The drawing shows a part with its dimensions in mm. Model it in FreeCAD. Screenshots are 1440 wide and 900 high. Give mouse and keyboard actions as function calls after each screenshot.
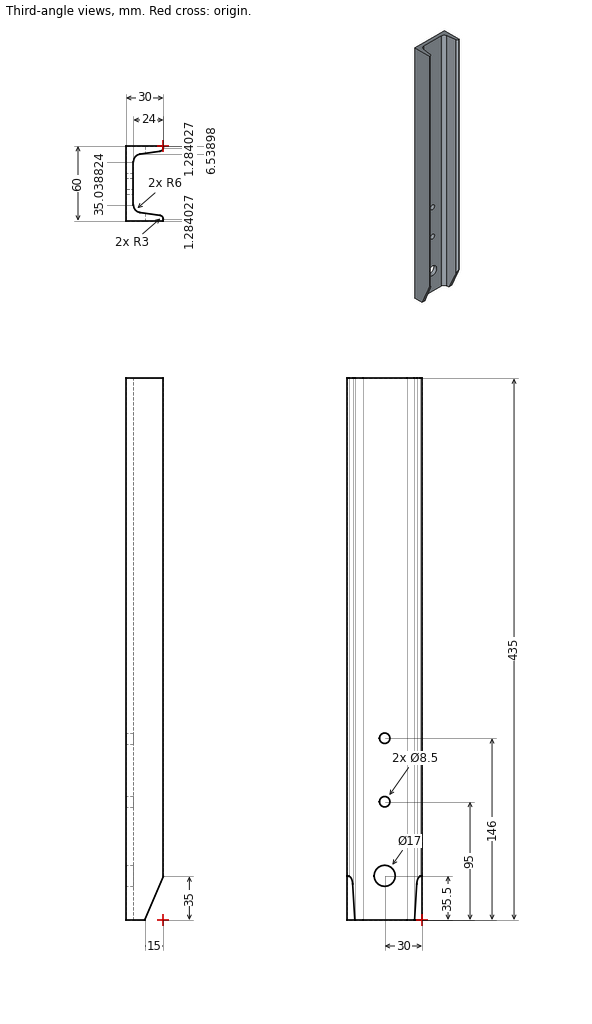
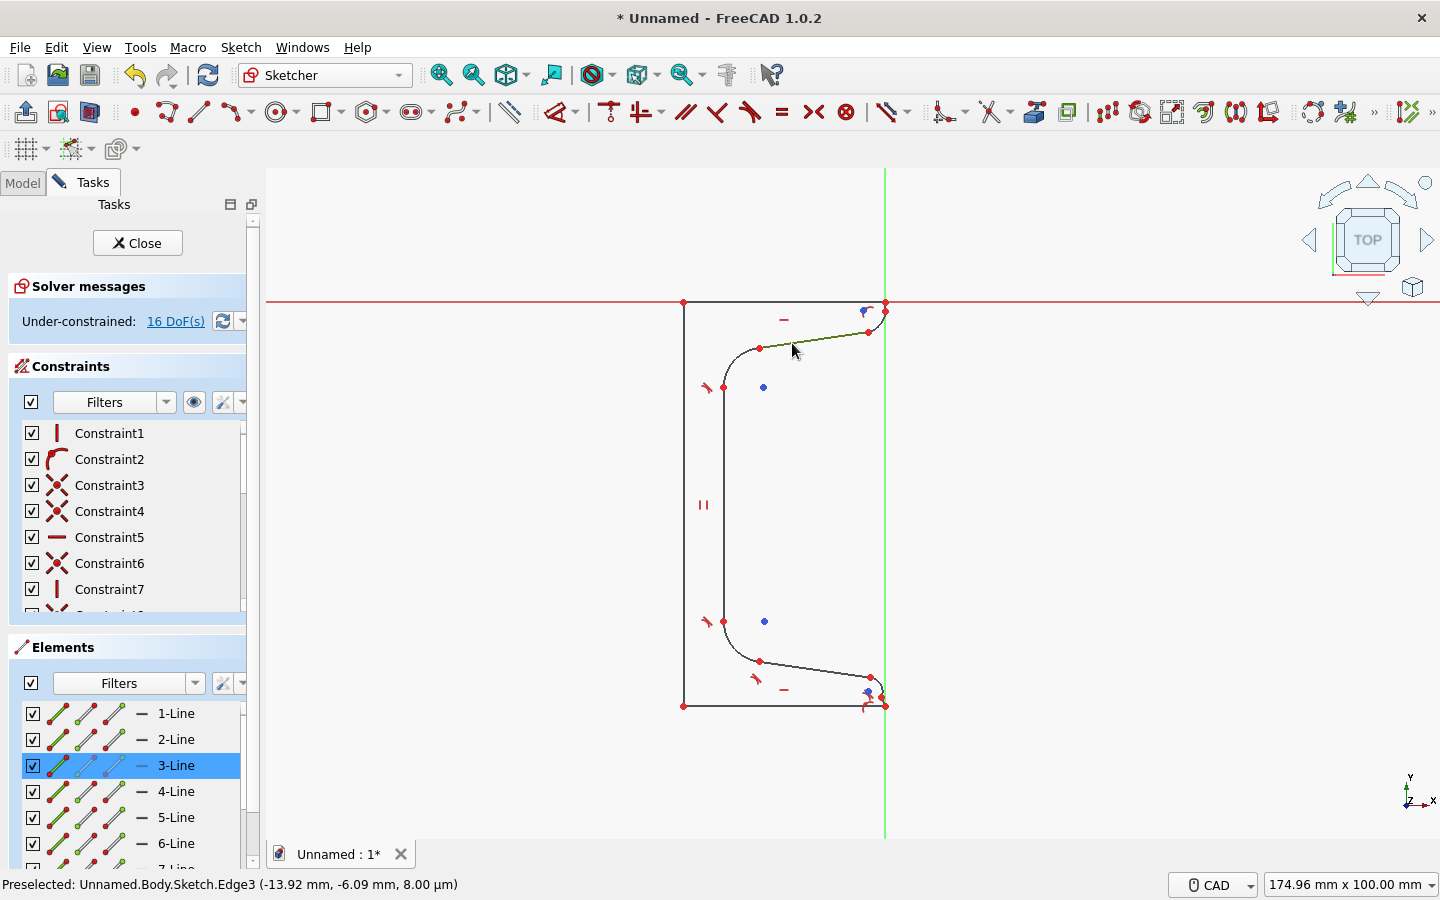
click(743, 353)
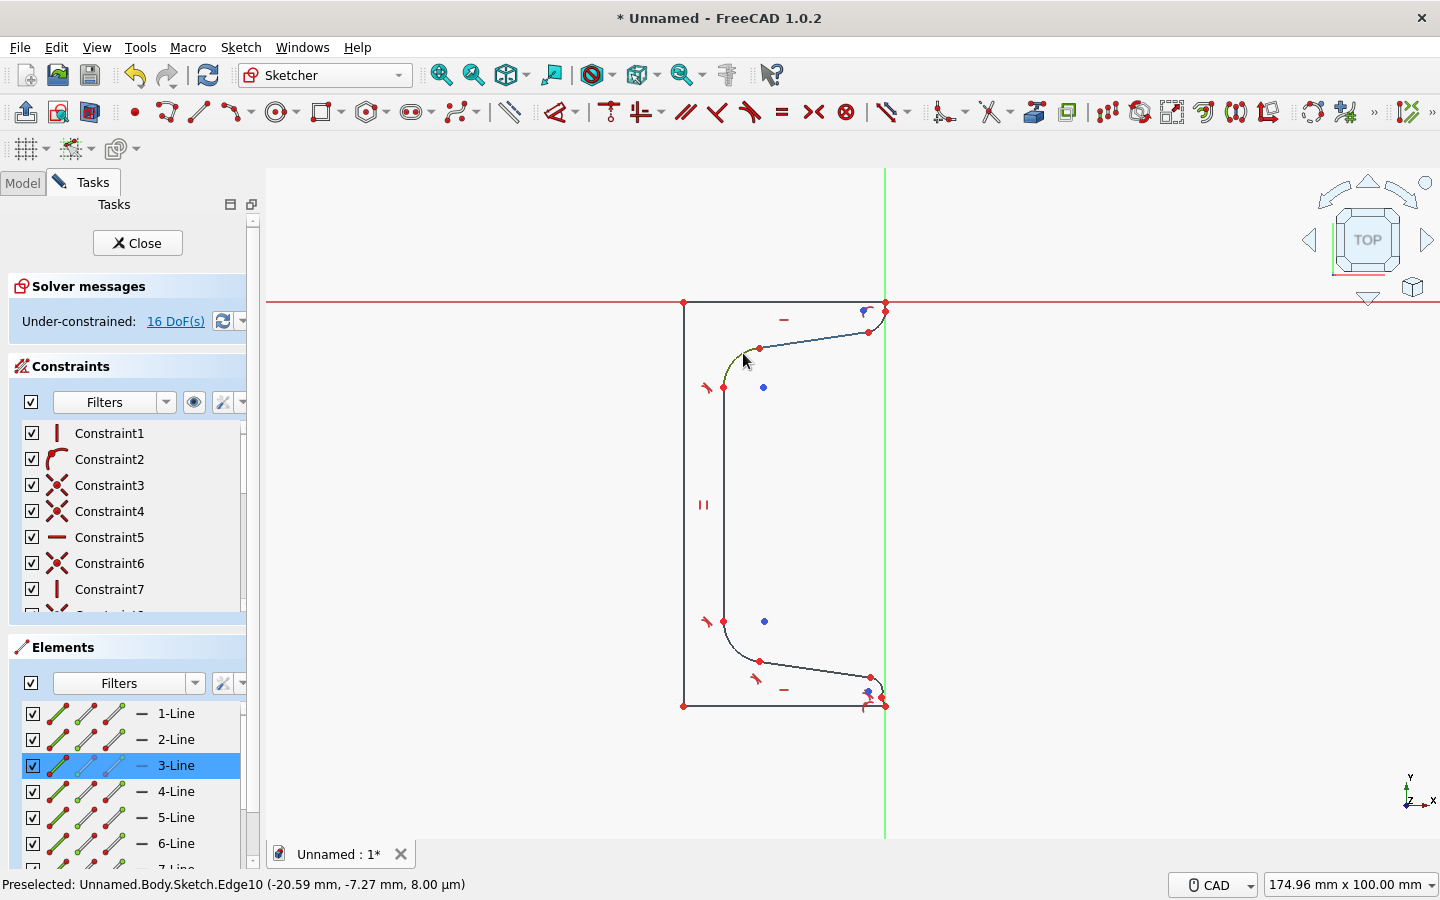
key(t)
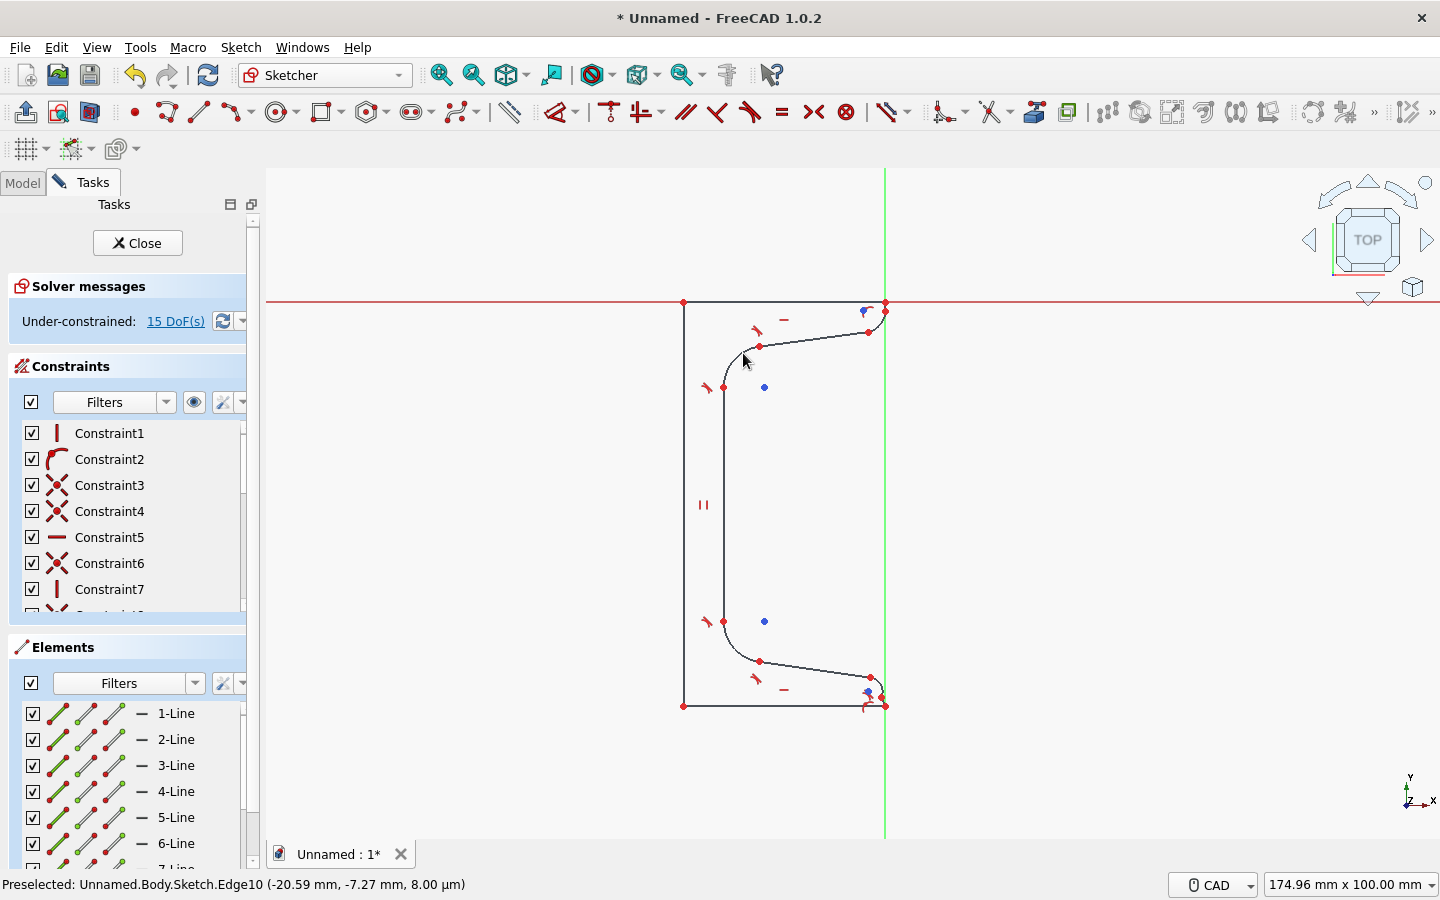
click(792, 342)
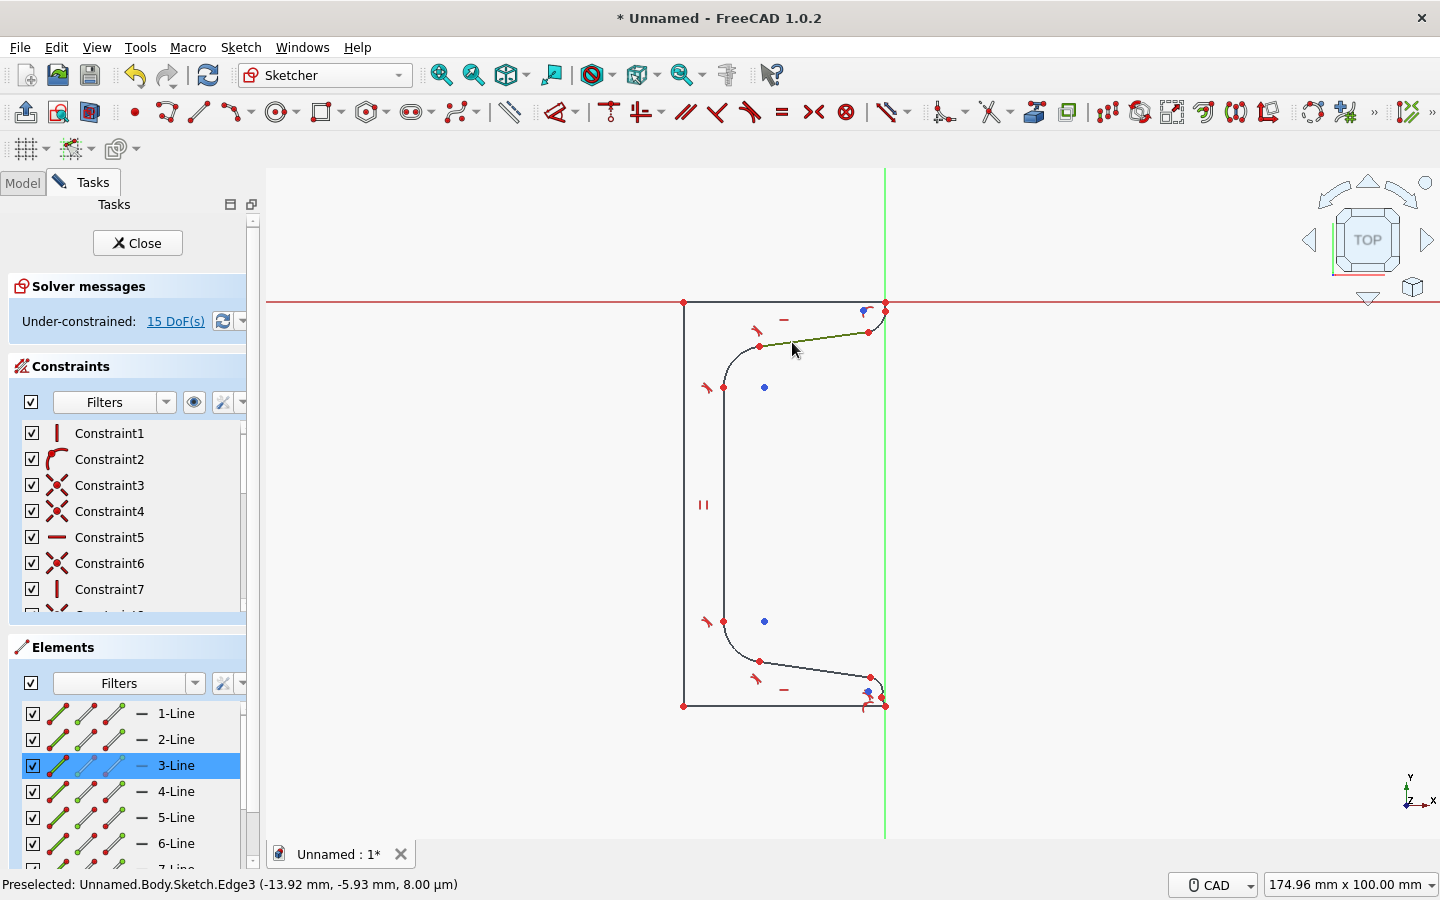
scroll(883, 320, up, 3)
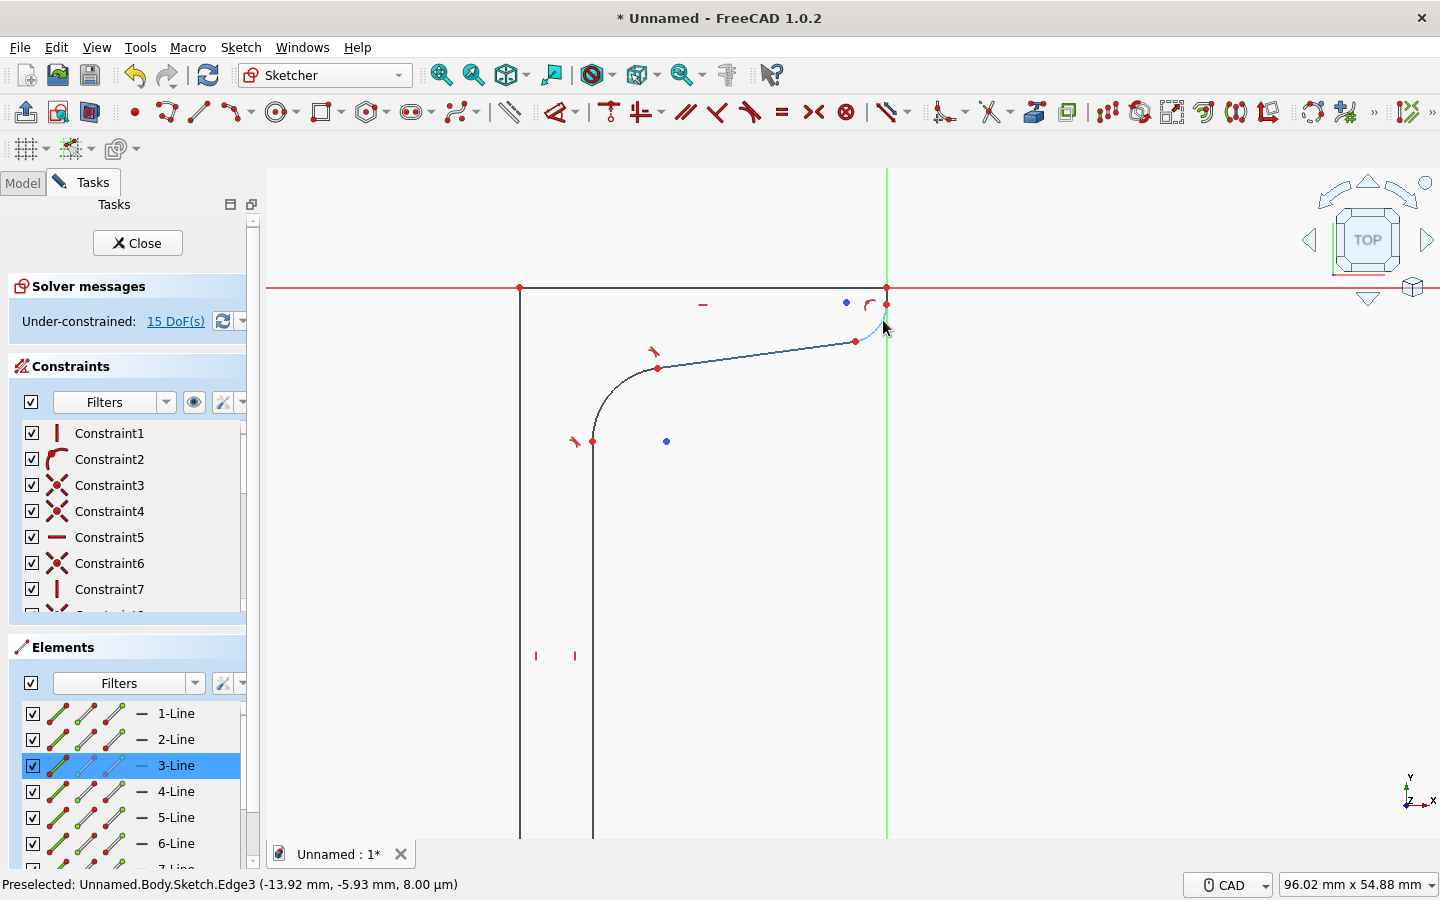
click(883, 320)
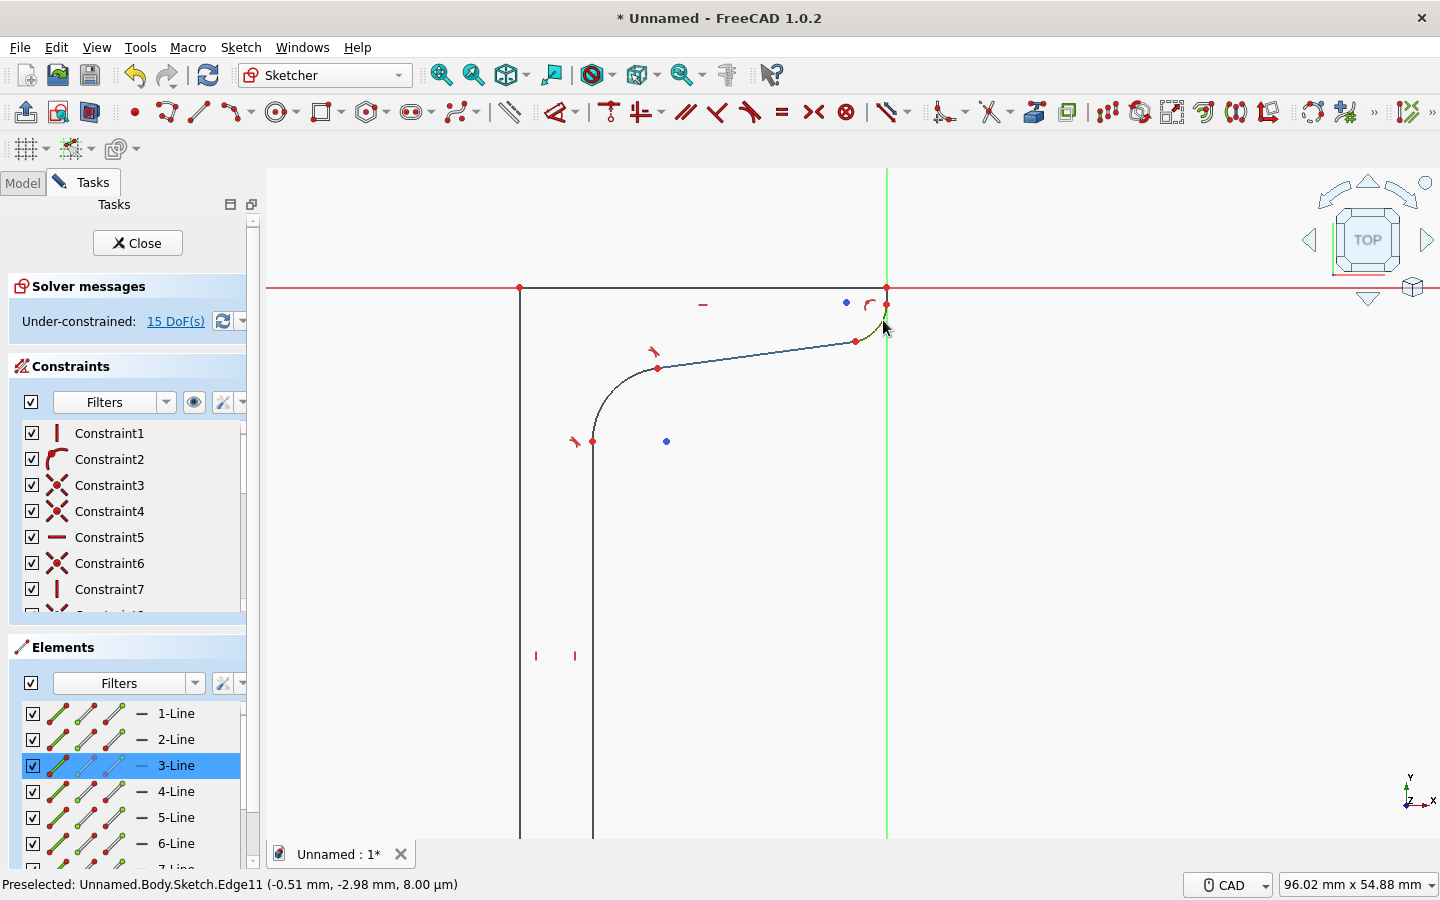
key(t)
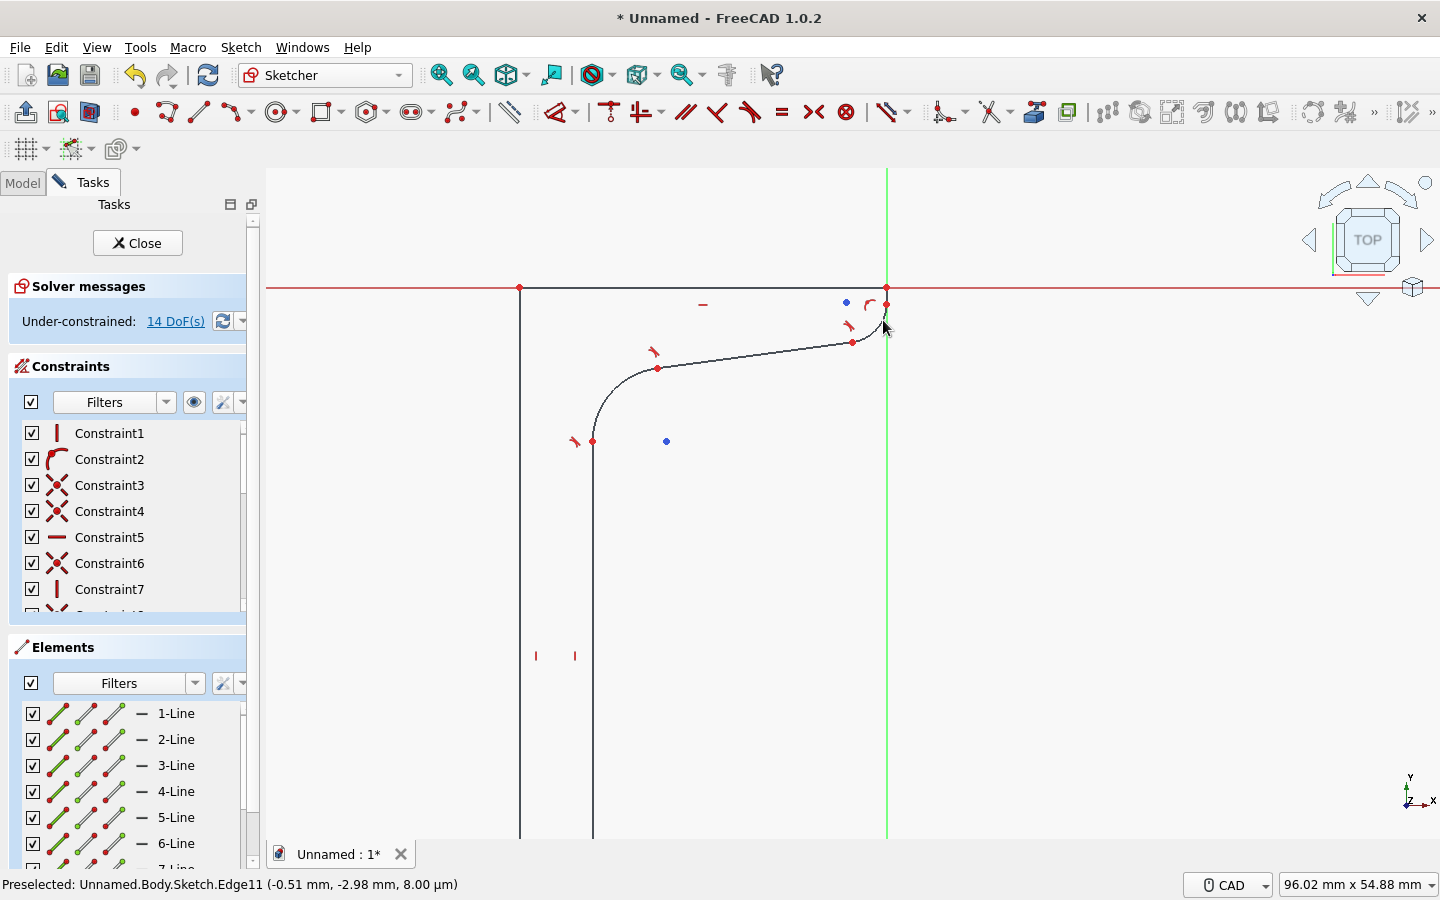
scroll(887, 296, up, 3)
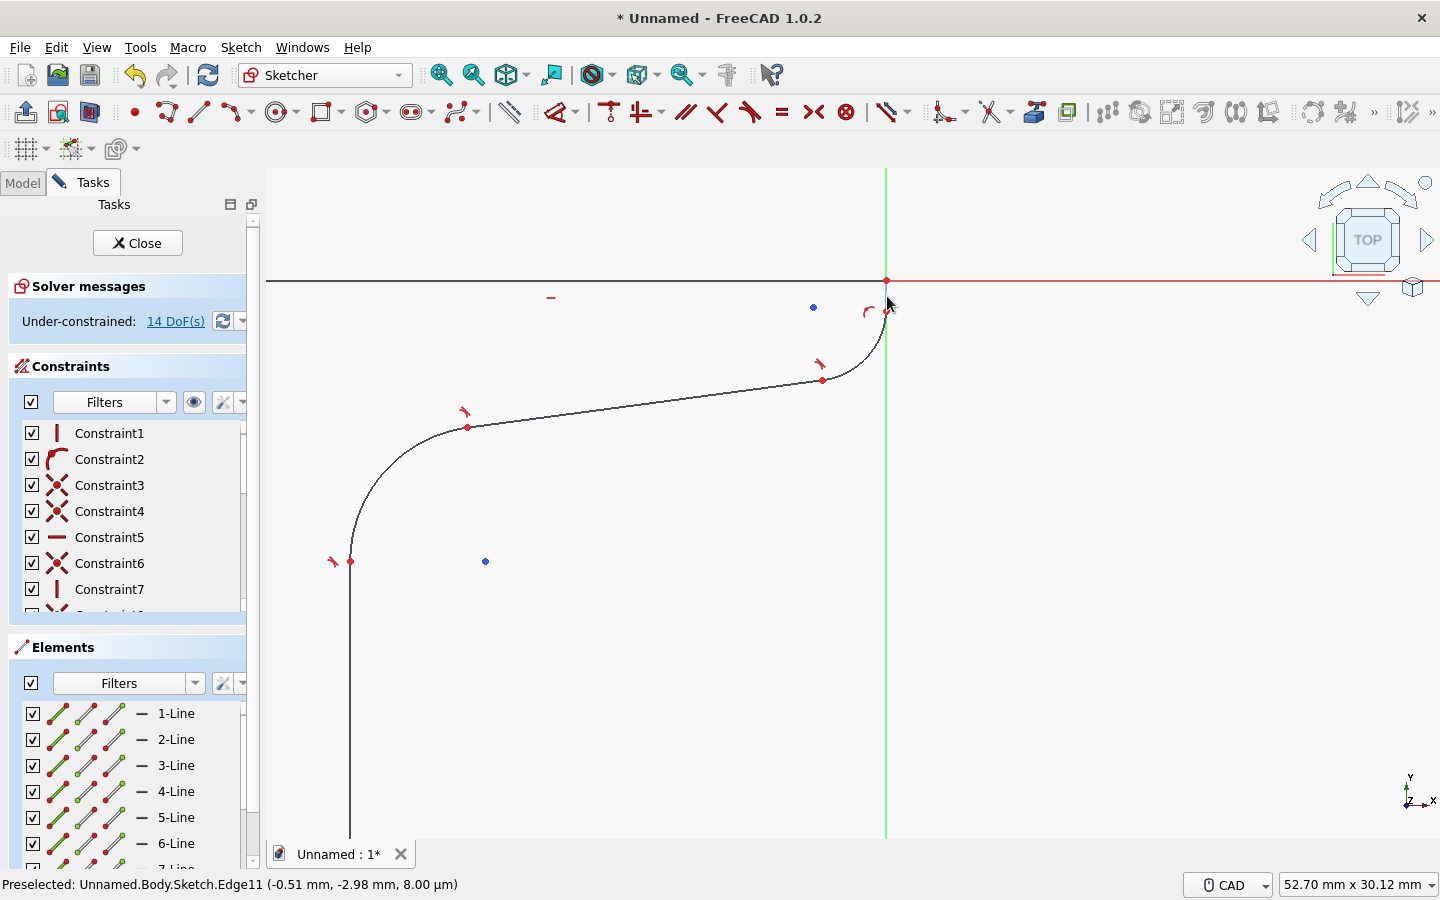
click(886, 296)